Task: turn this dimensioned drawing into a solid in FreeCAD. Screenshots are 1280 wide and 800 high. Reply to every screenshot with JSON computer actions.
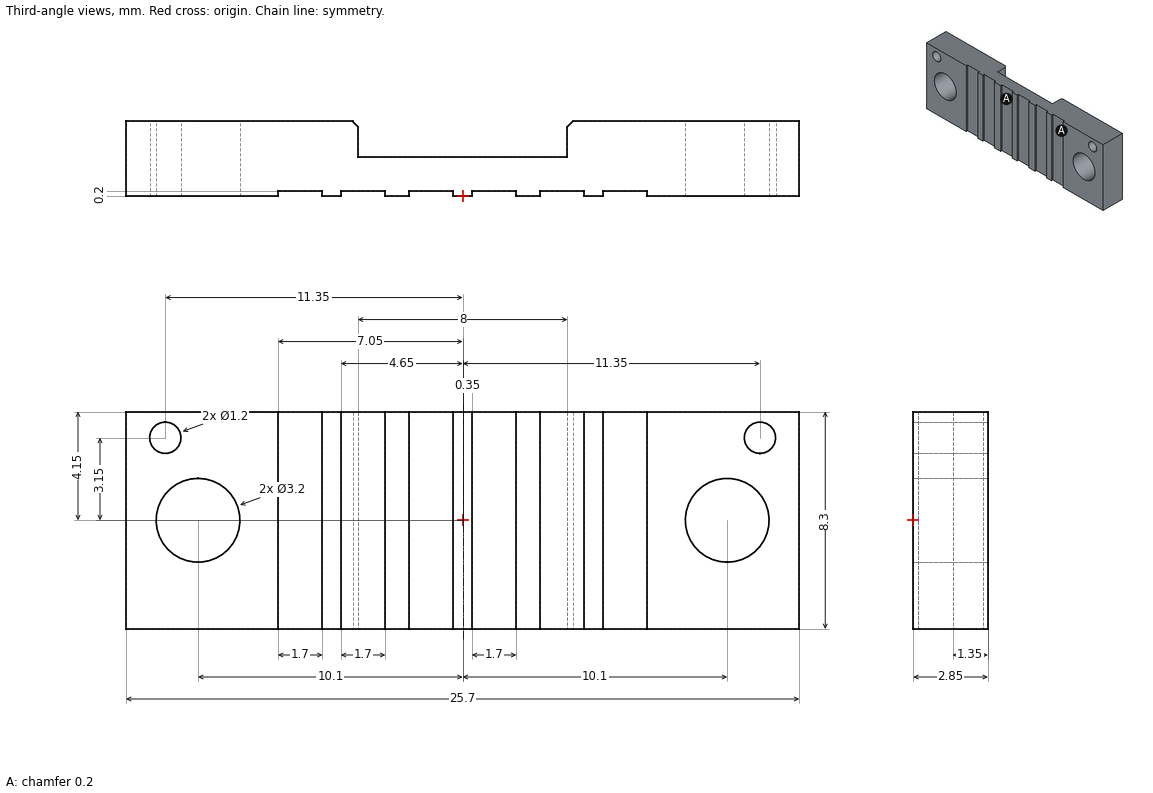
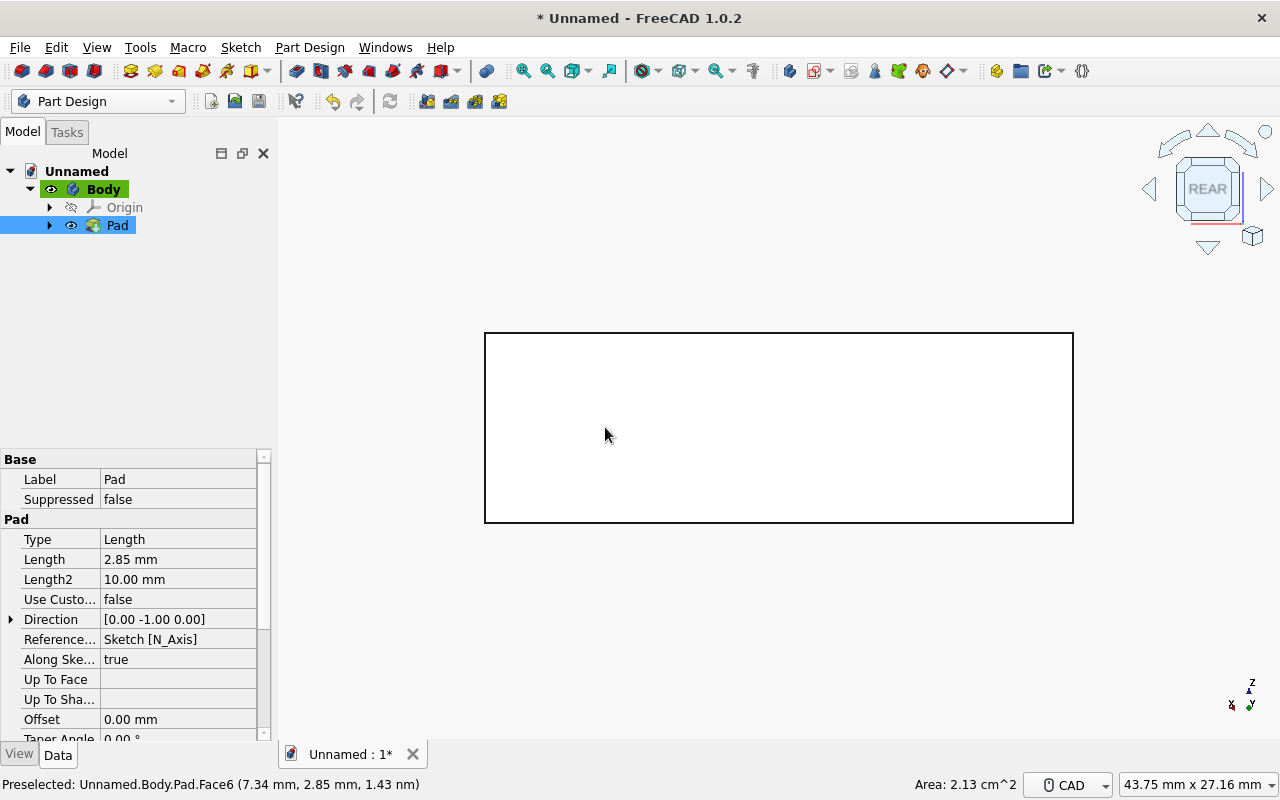
{"action": "left_click", "coordinate": [814, 72]}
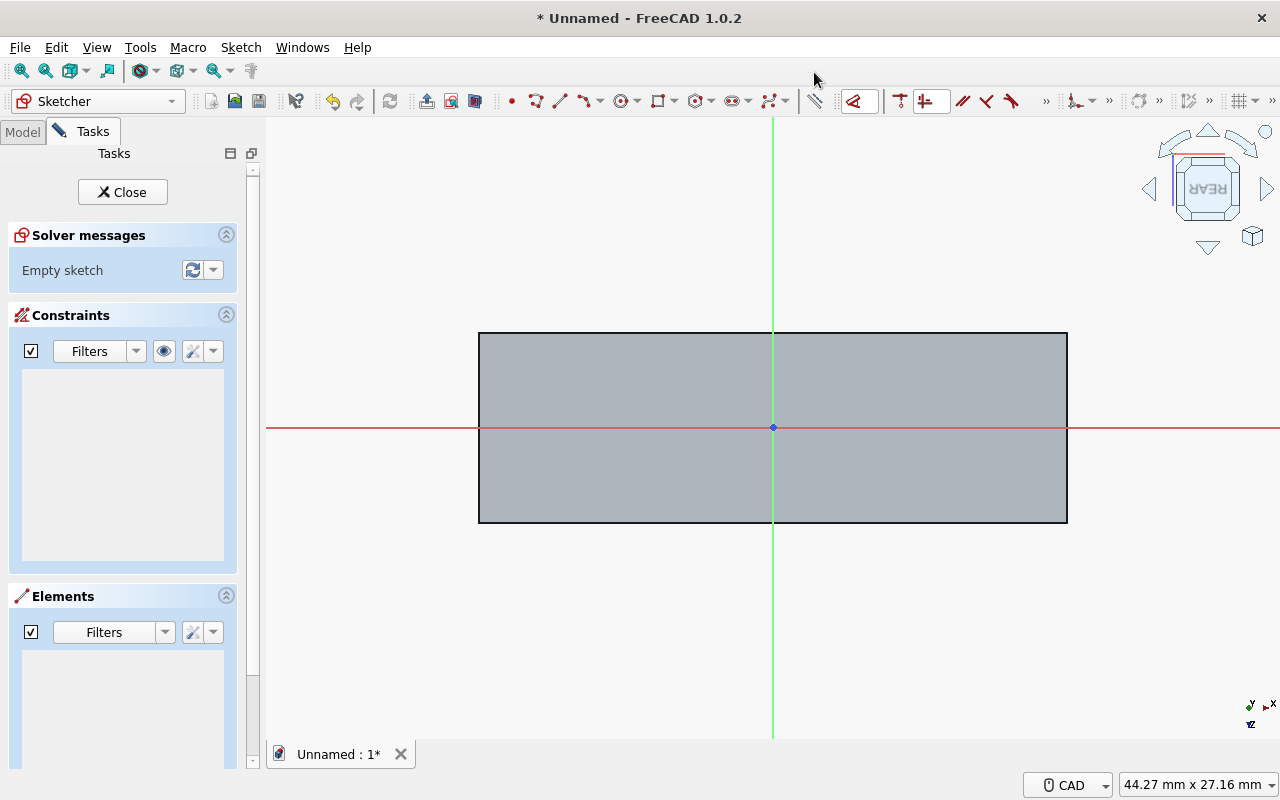
{"action": "key", "text": "g c"}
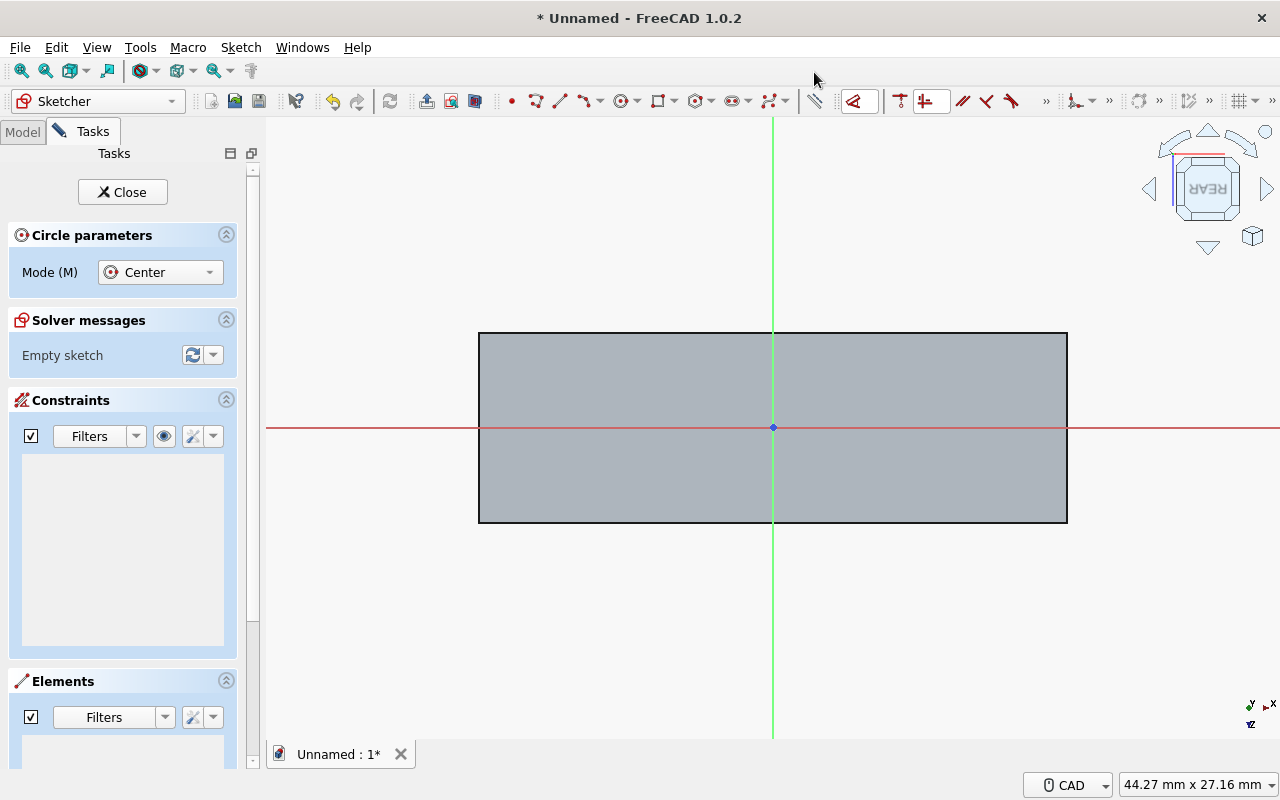
{"action": "left_click", "coordinate": [542, 428]}
{"action": "left_click", "coordinate": [568, 402]}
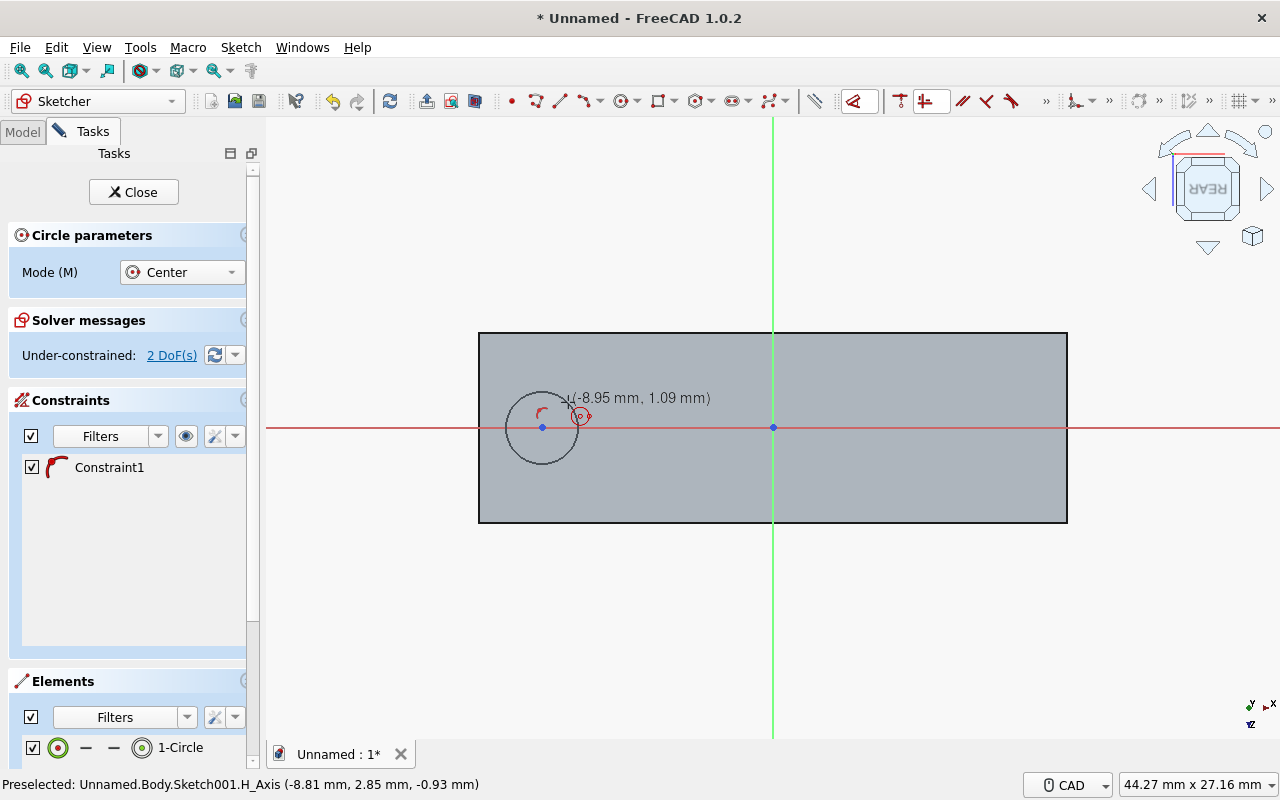
{"action": "scroll", "coordinate": [513, 500], "scroll_direction": "up", "scroll_amount": 3}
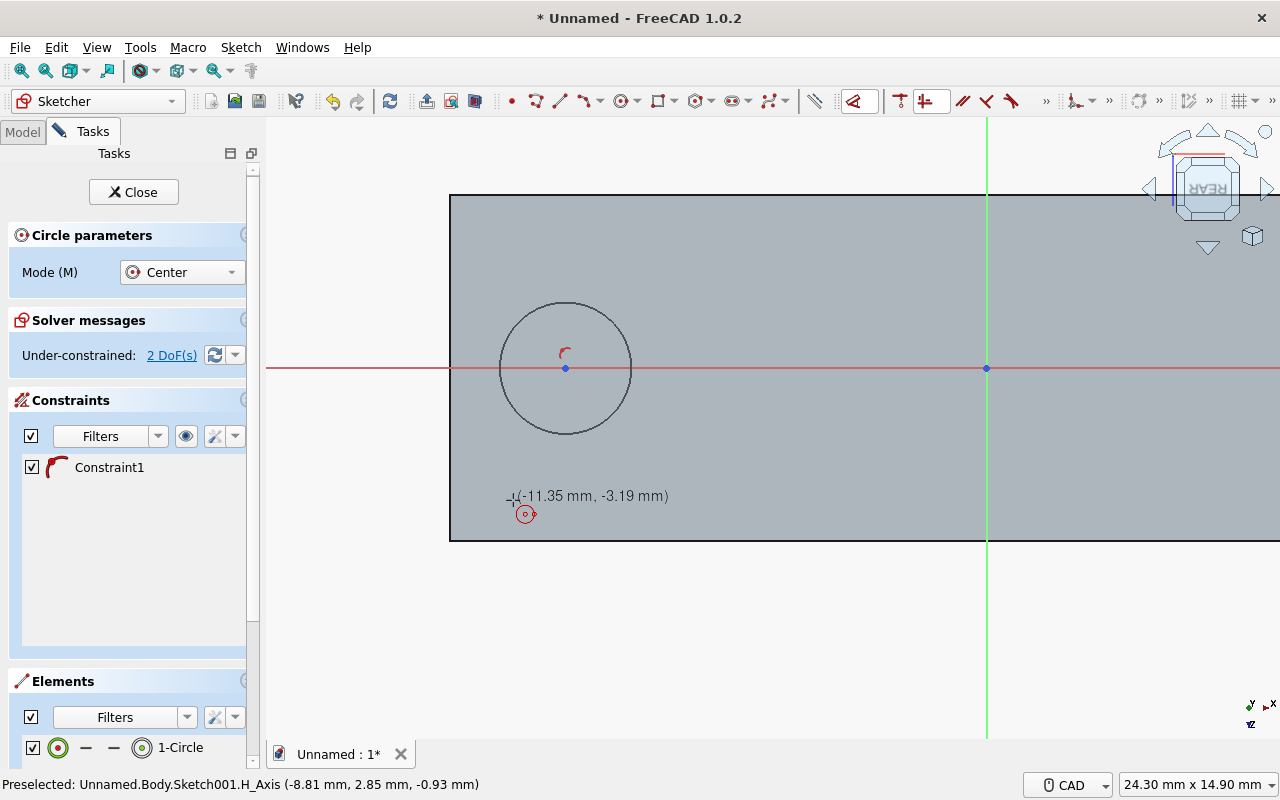
{"action": "left_click", "coordinate": [513, 500]}
{"action": "left_click", "coordinate": [531, 482]}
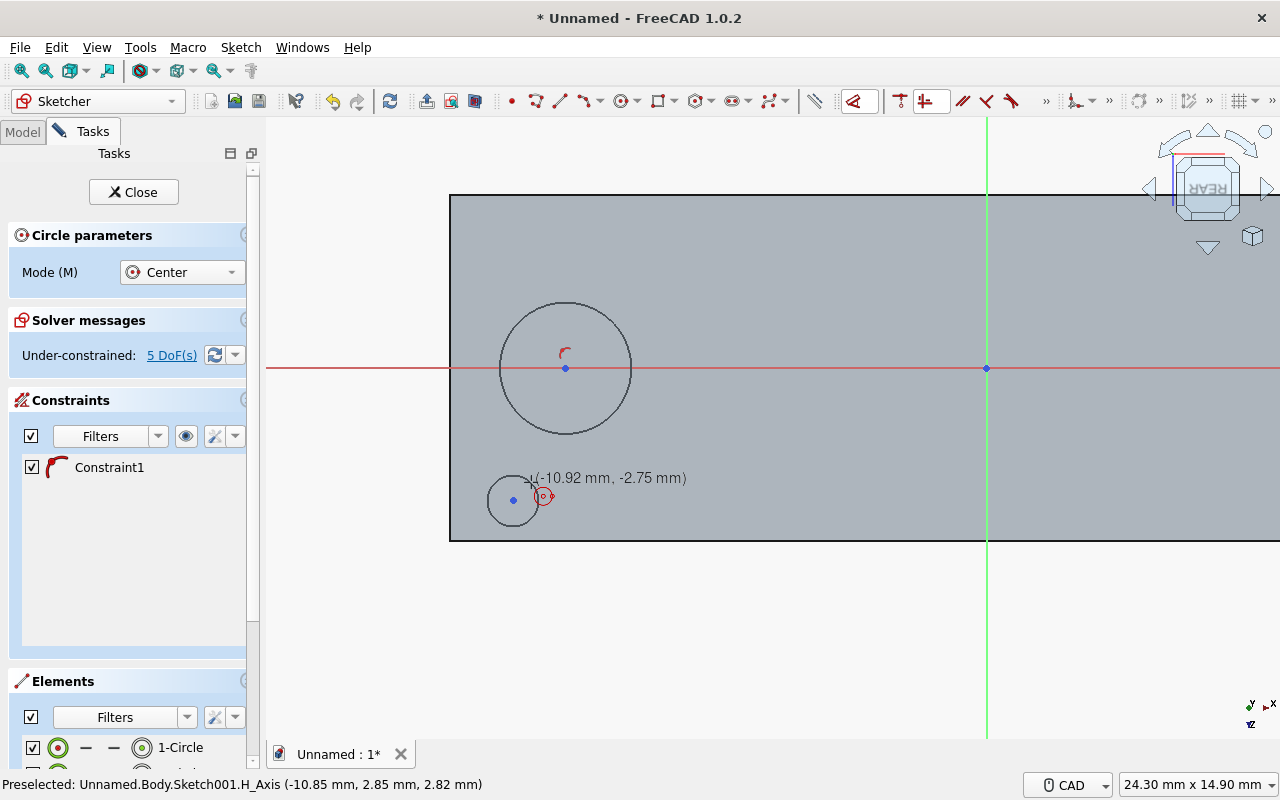
{"action": "scroll", "coordinate": [361, 446], "scroll_direction": "down", "scroll_amount": 3}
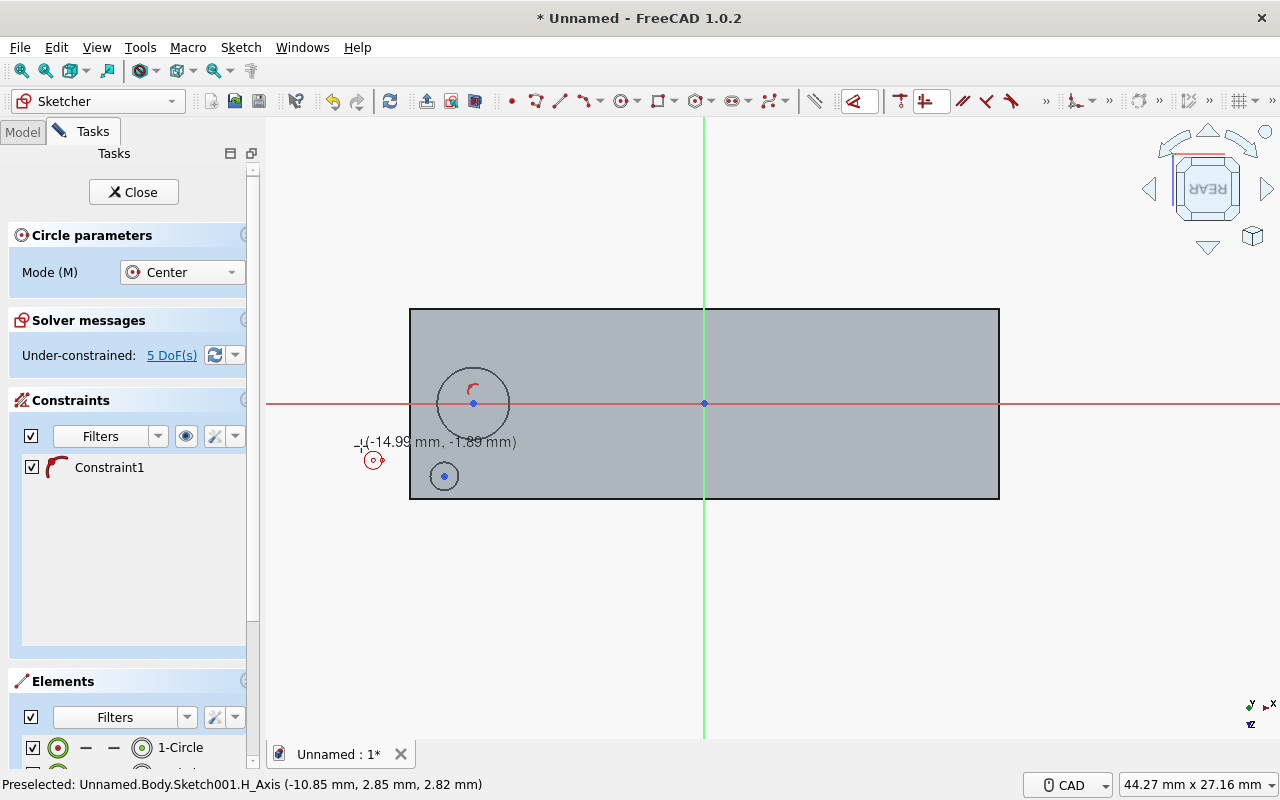
{"action": "left_click", "coordinate": [936, 404]}
{"action": "left_click", "coordinate": [962, 378]}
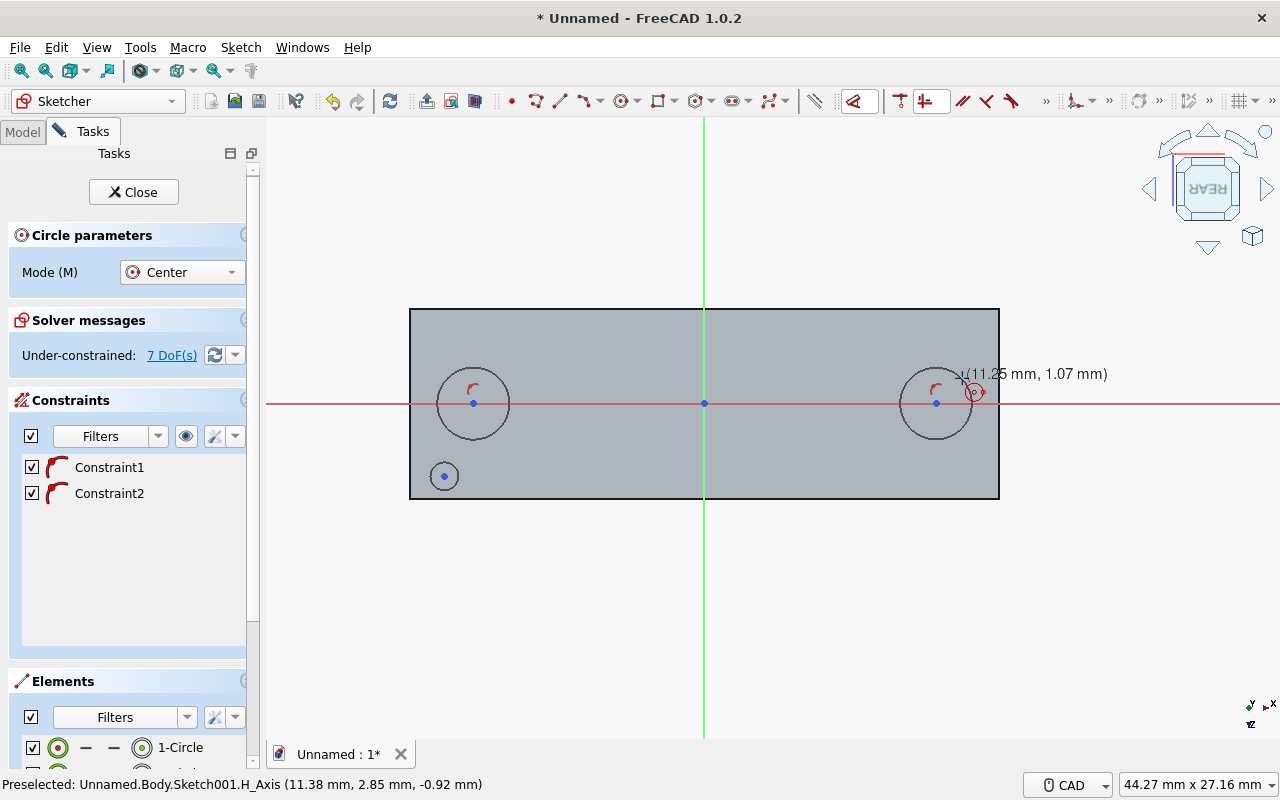
{"action": "scroll", "coordinate": [964, 476], "scroll_direction": "up", "scroll_amount": 3}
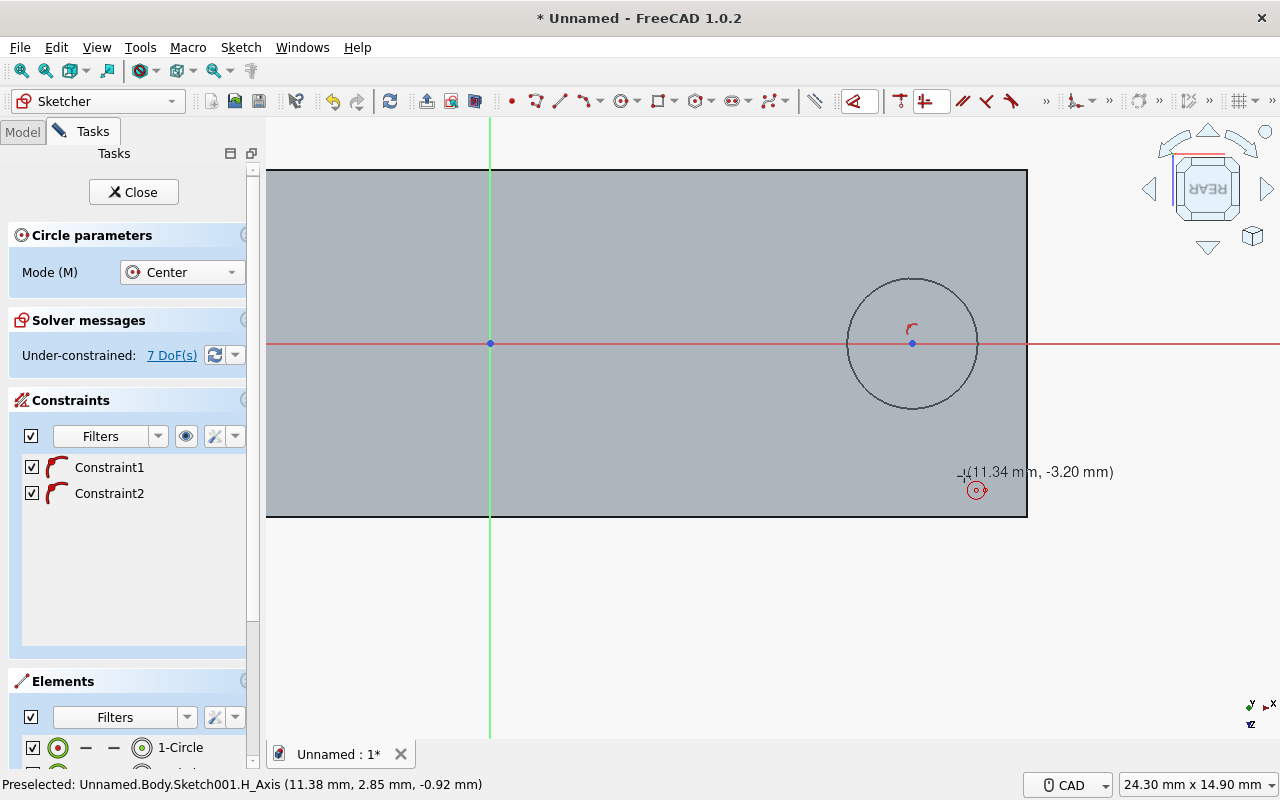
{"action": "left_click", "coordinate": [964, 475]}
{"action": "left_click", "coordinate": [982, 457]}
{"action": "key", "text": "Escape"}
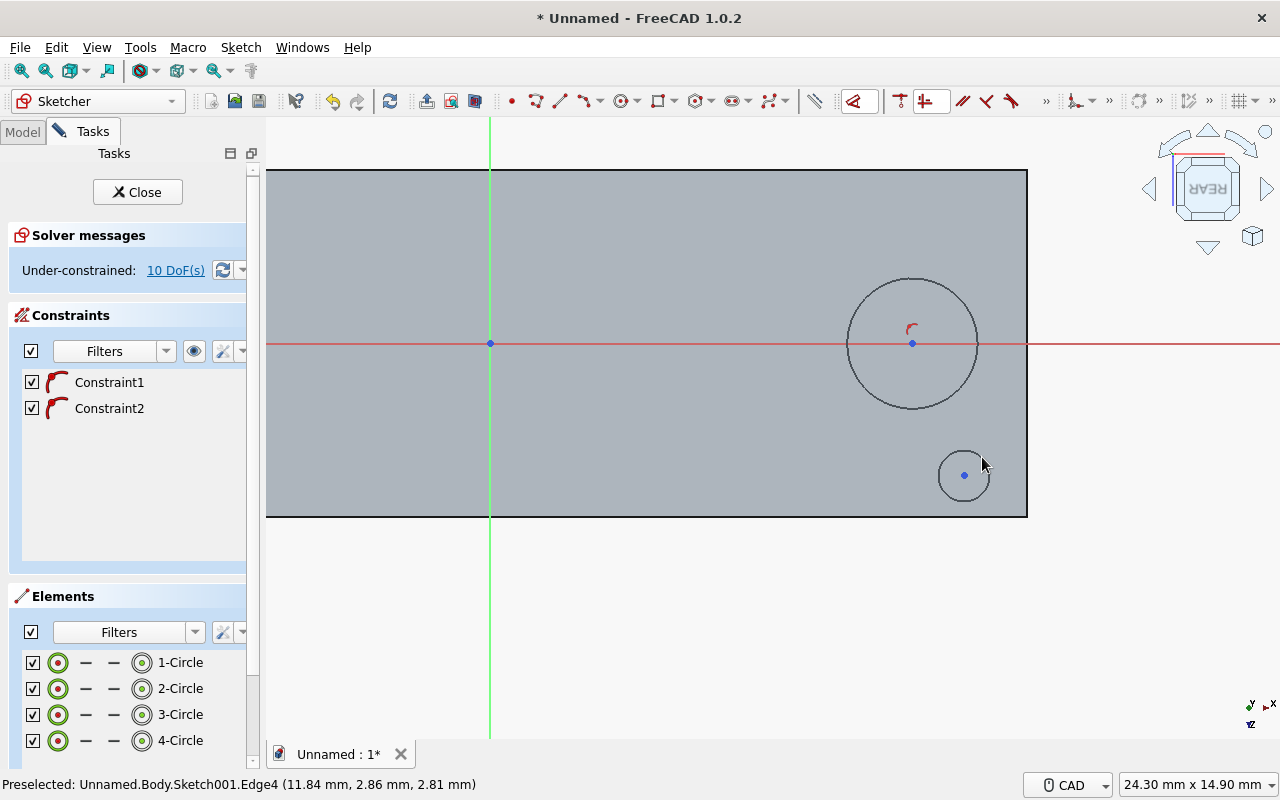
{"action": "scroll", "coordinate": [965, 476], "scroll_direction": "down", "scroll_amount": 3}